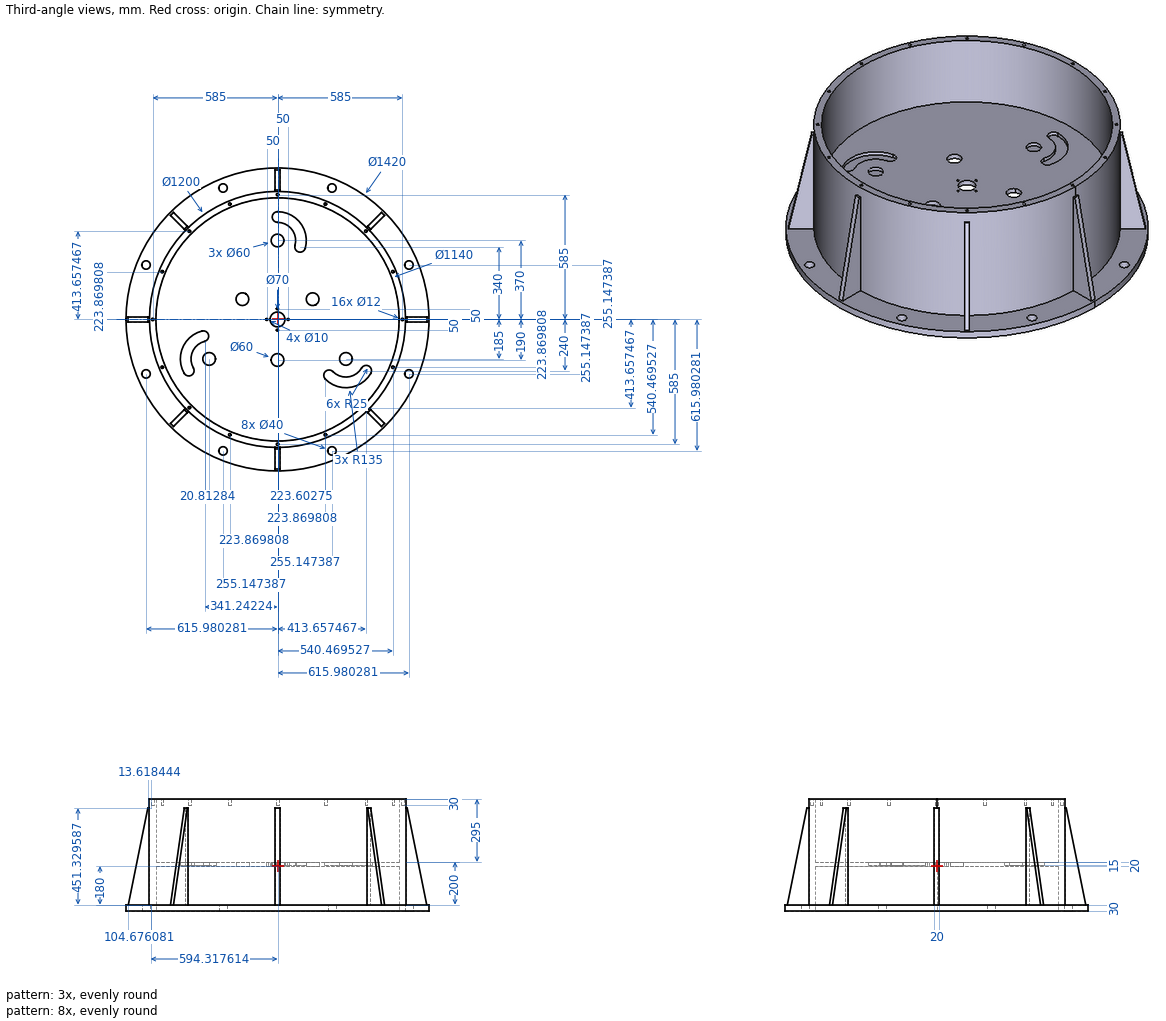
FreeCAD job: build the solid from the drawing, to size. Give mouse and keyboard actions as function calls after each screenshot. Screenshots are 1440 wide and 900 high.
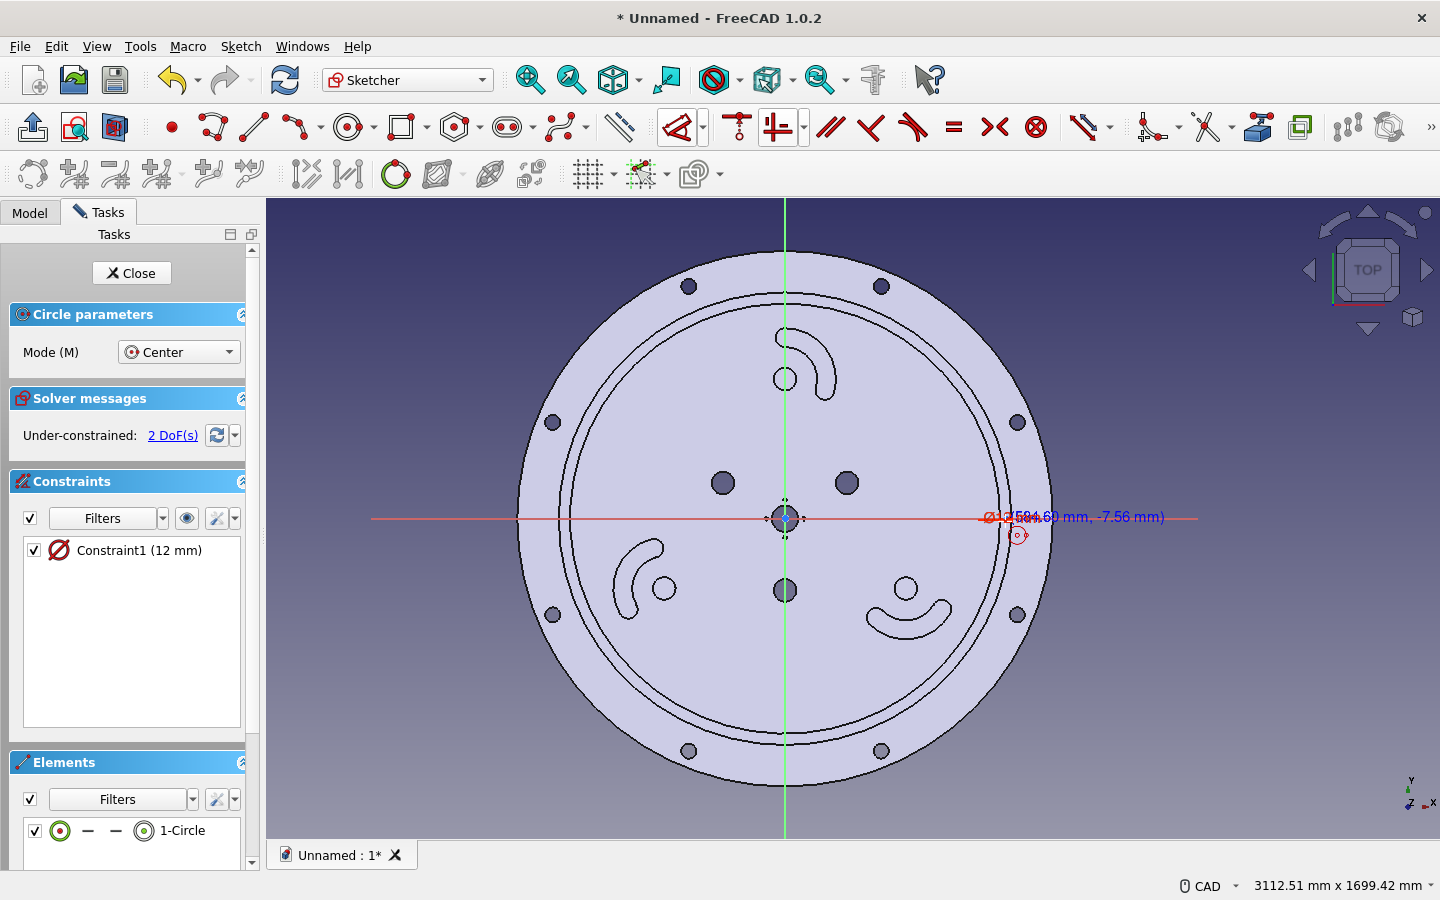
scroll(989, 603, up, 12)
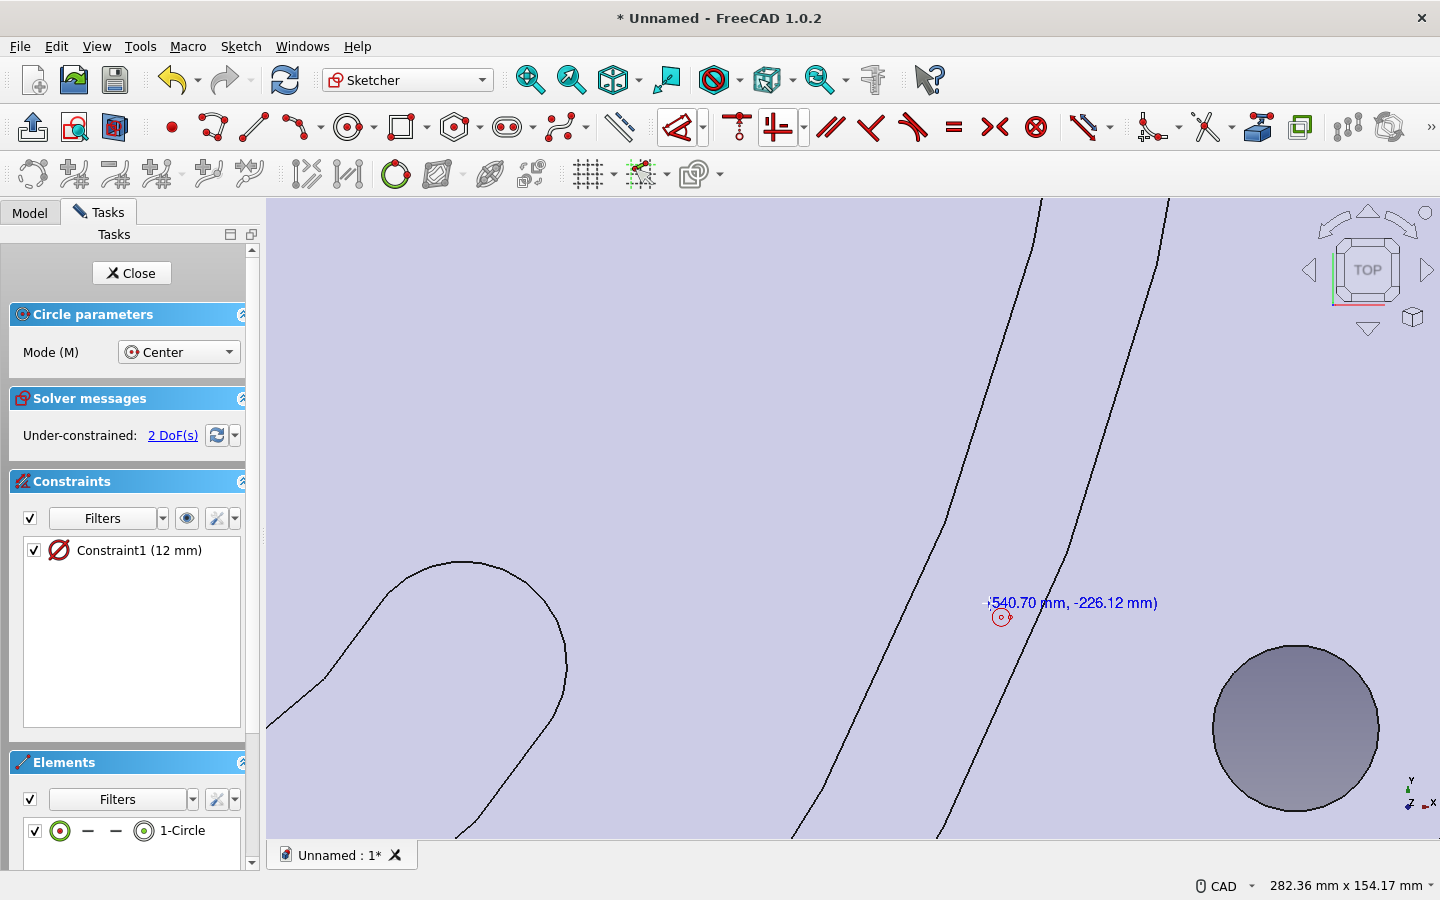
scroll(989, 603, down, 12)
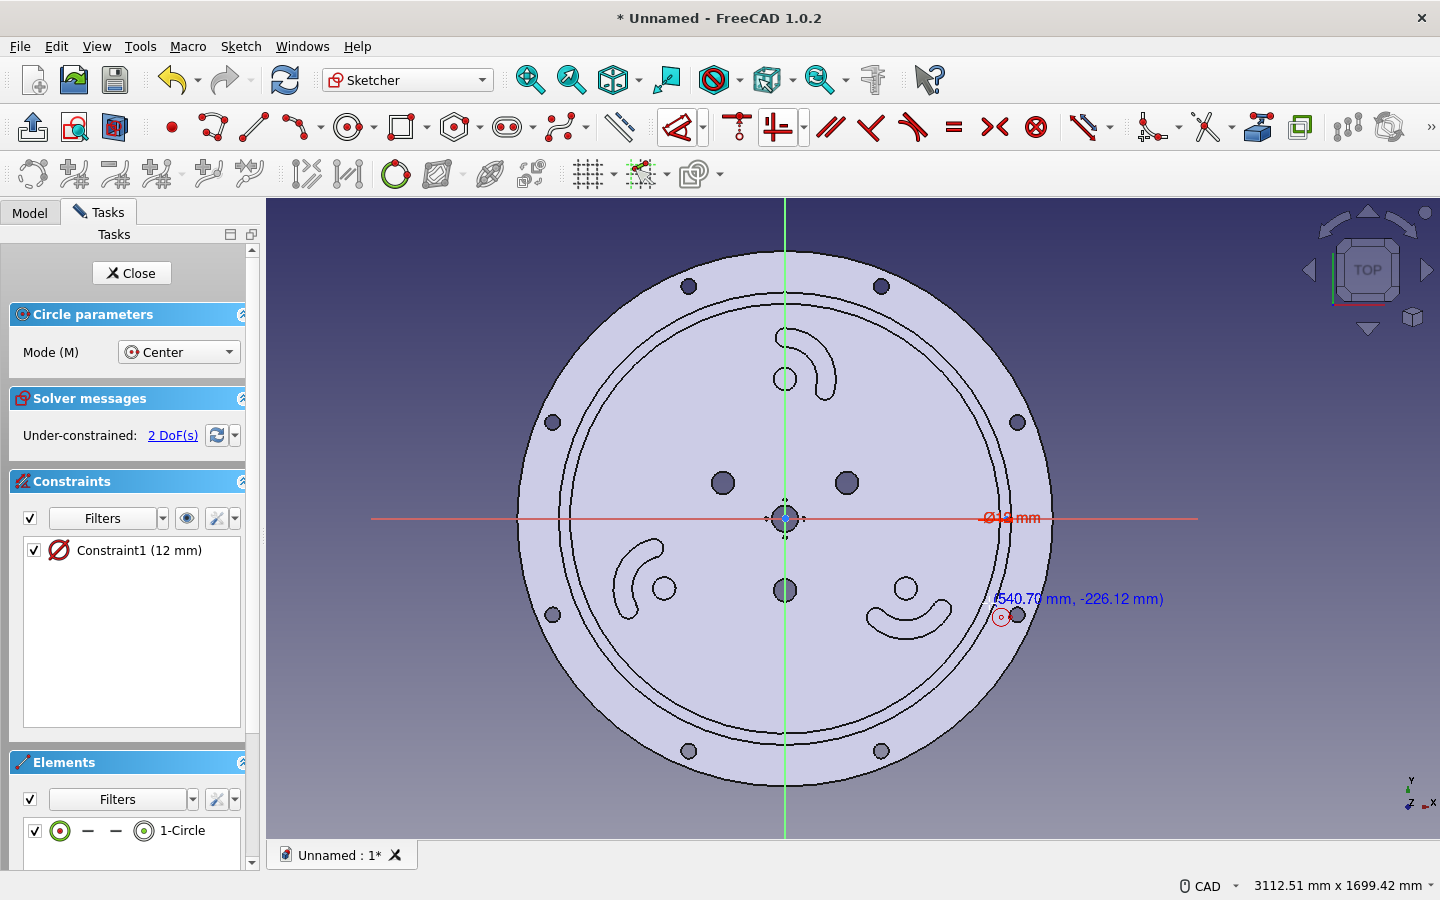
click(989, 603)
move(991, 602)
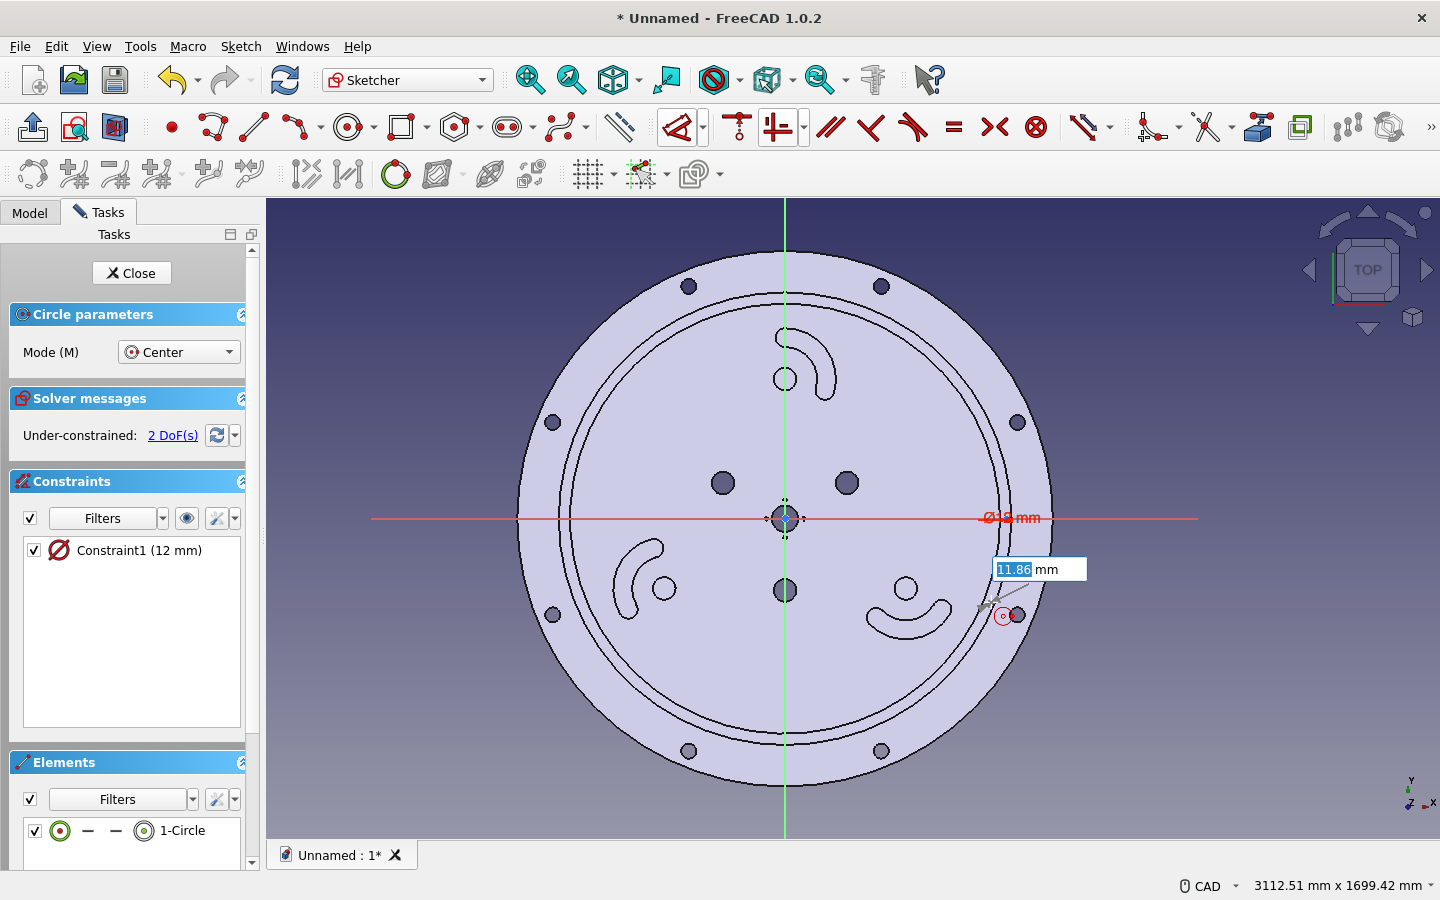
text(12)
key(Return)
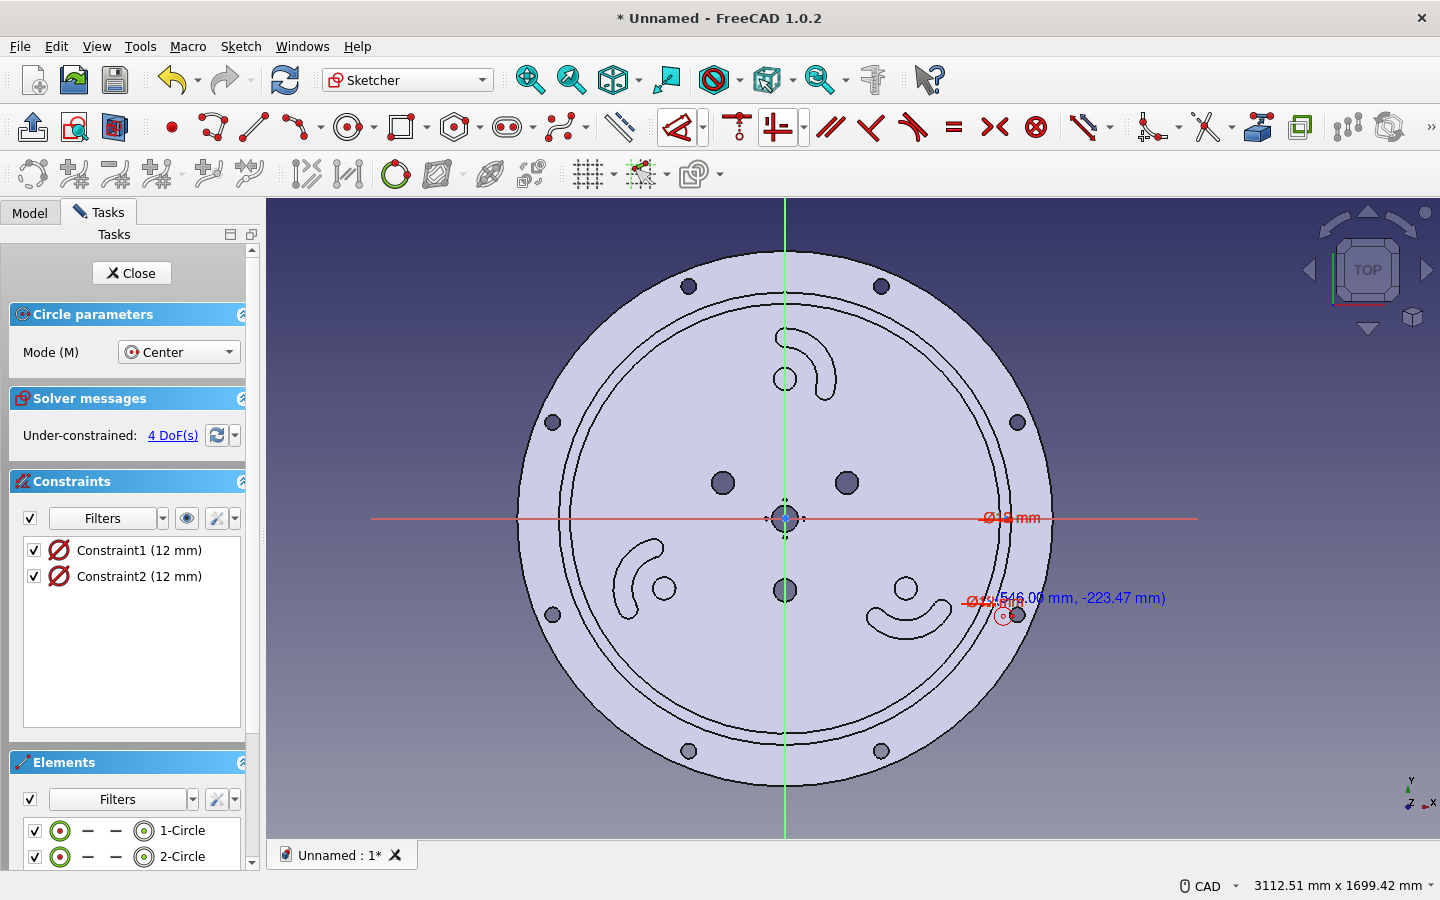
scroll(941, 675, up, 12)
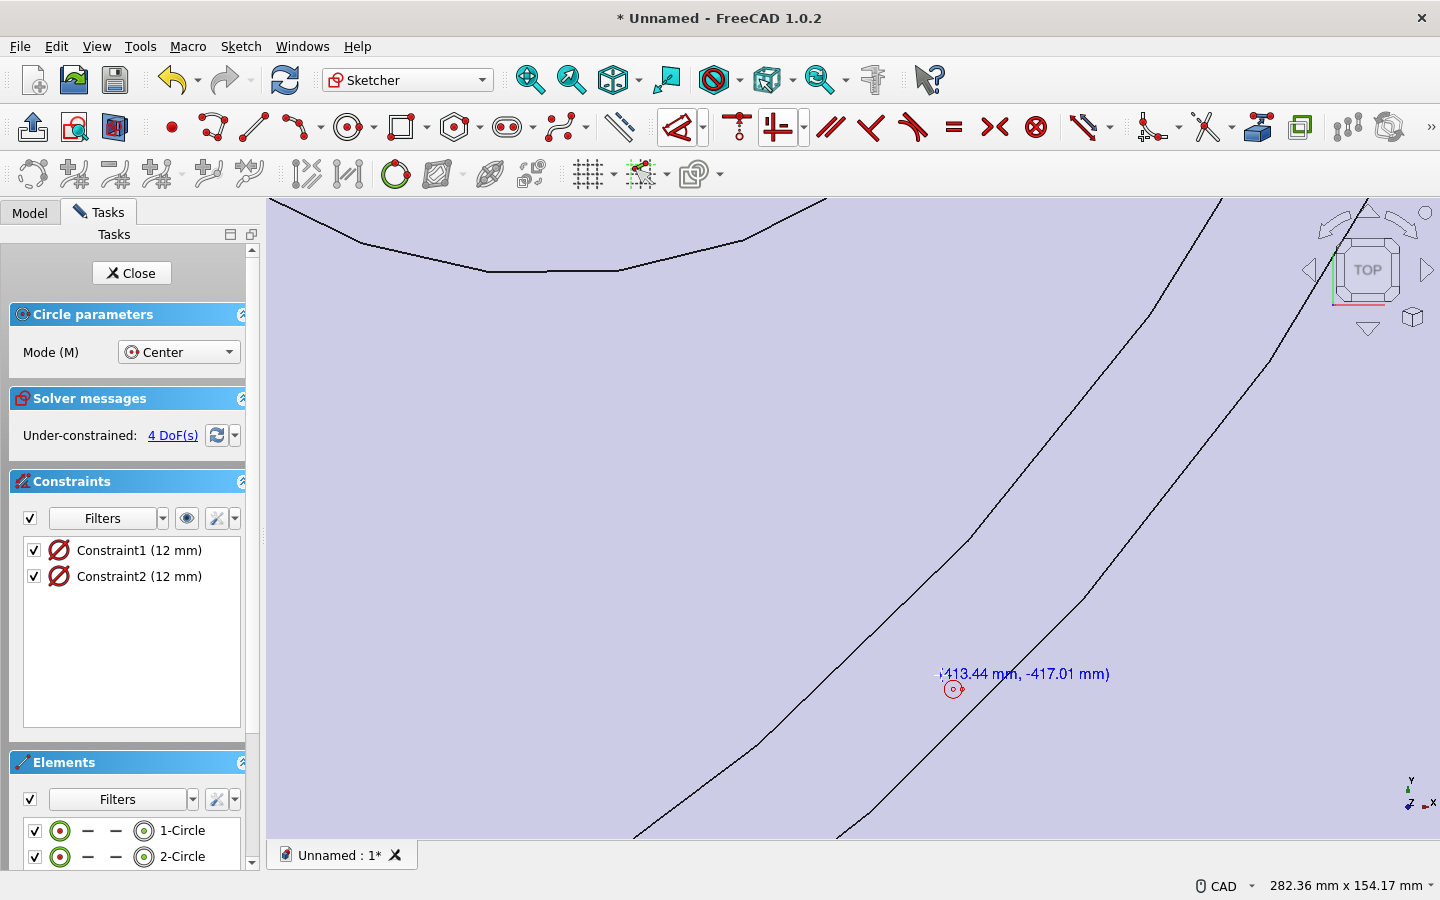
scroll(941, 676, down, 12)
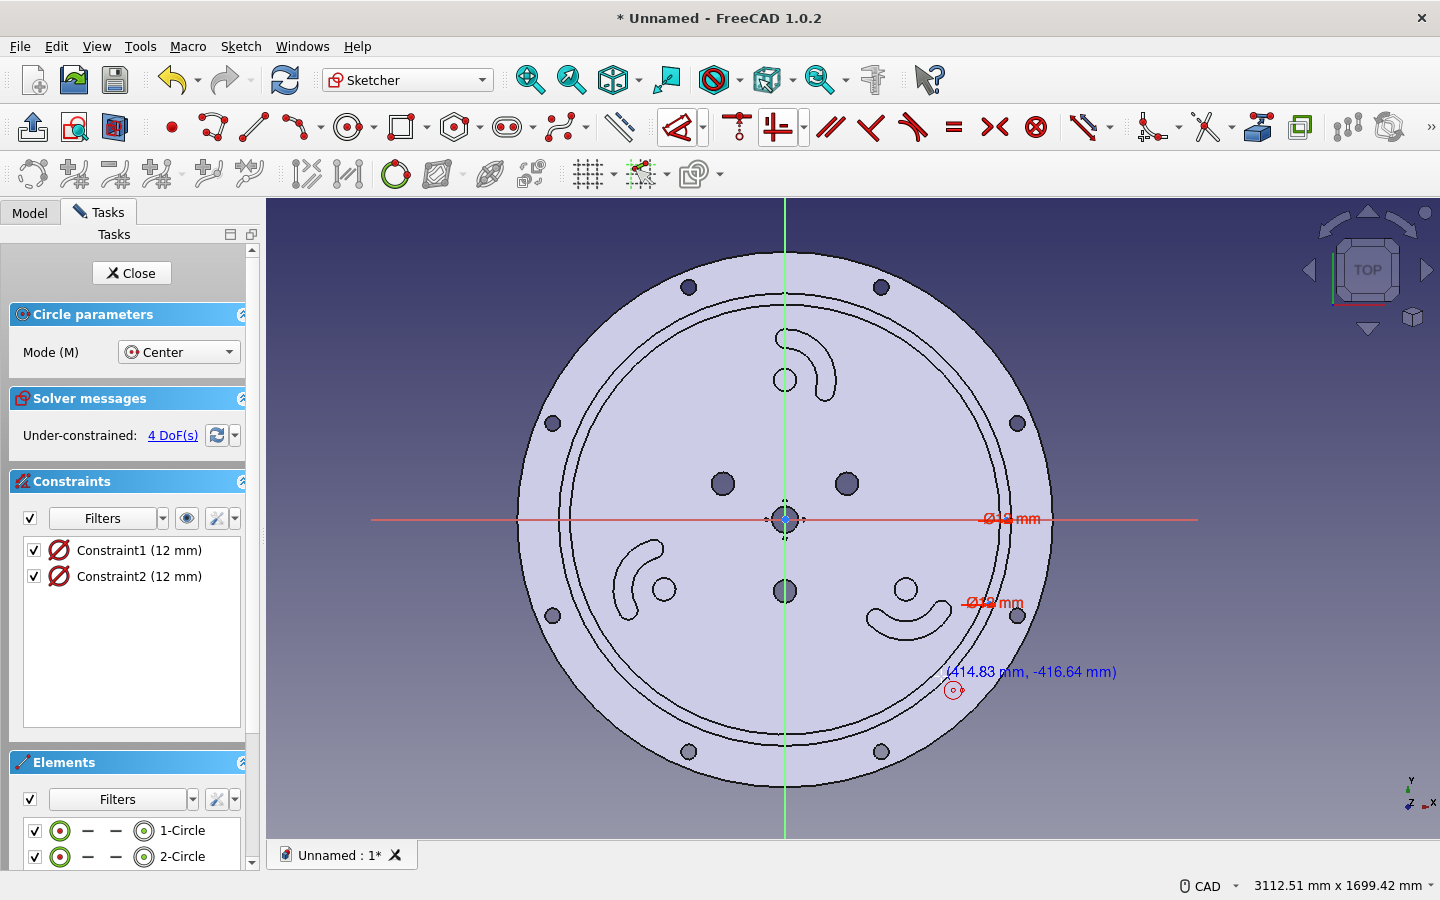
click(941, 676)
move(943, 674)